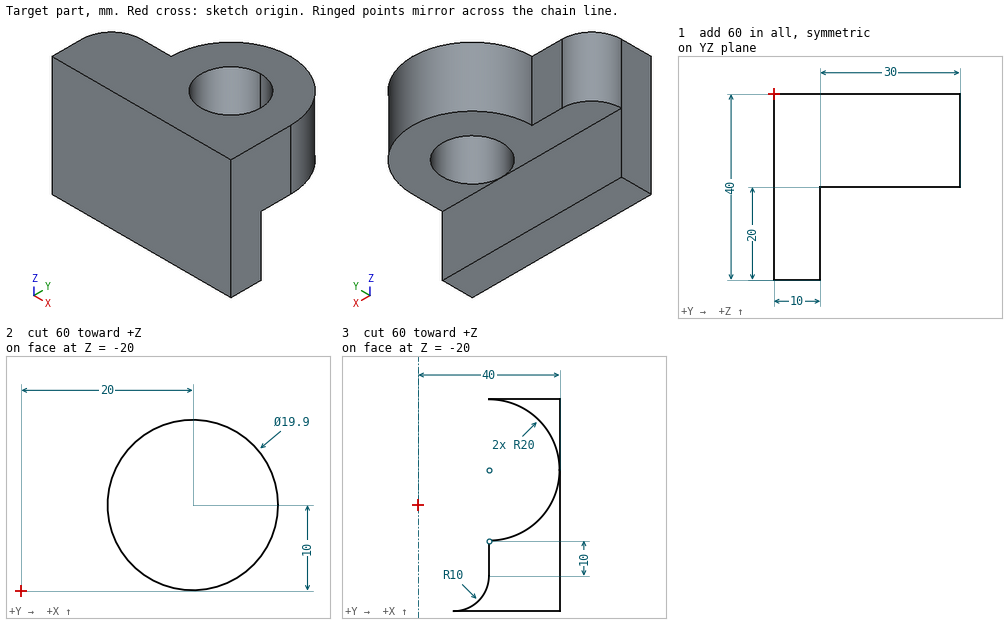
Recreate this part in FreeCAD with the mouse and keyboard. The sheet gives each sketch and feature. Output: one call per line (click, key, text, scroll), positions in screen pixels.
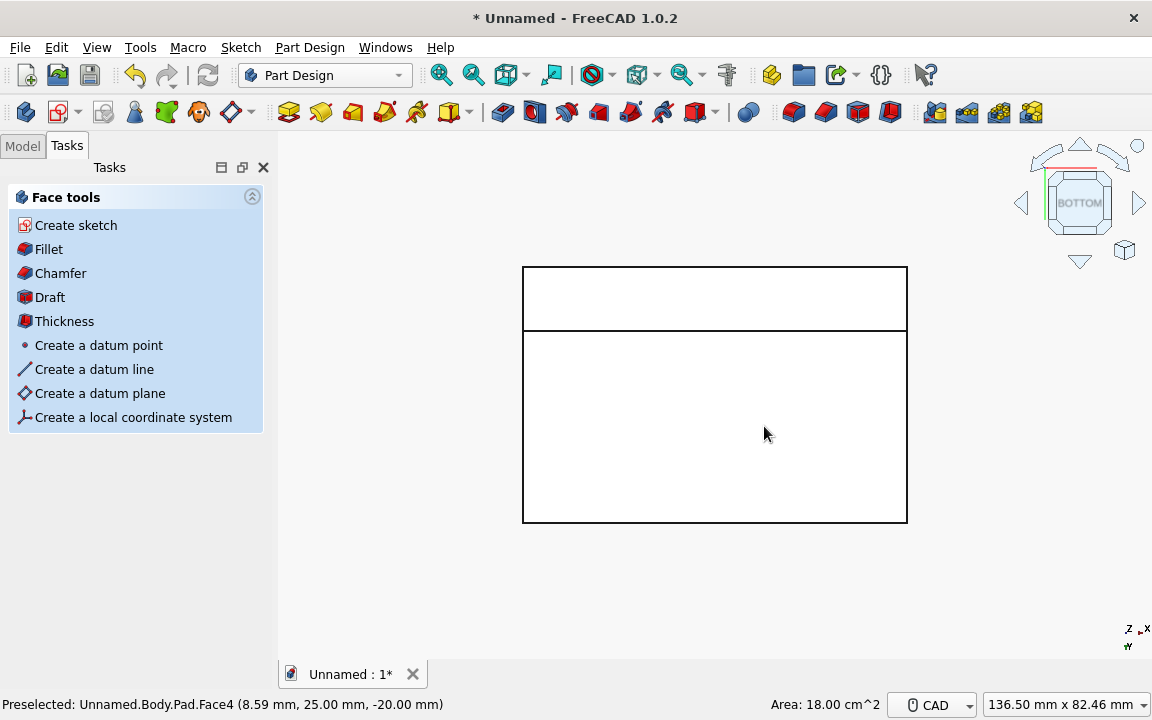
click(58, 112)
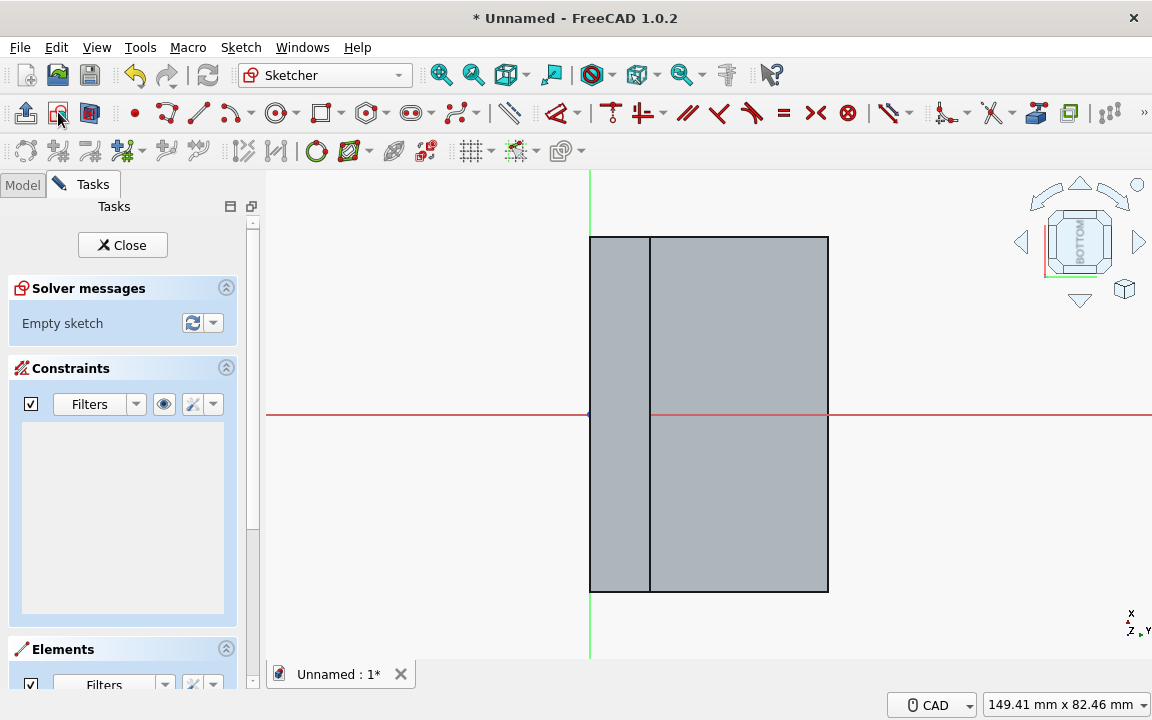
click(90, 114)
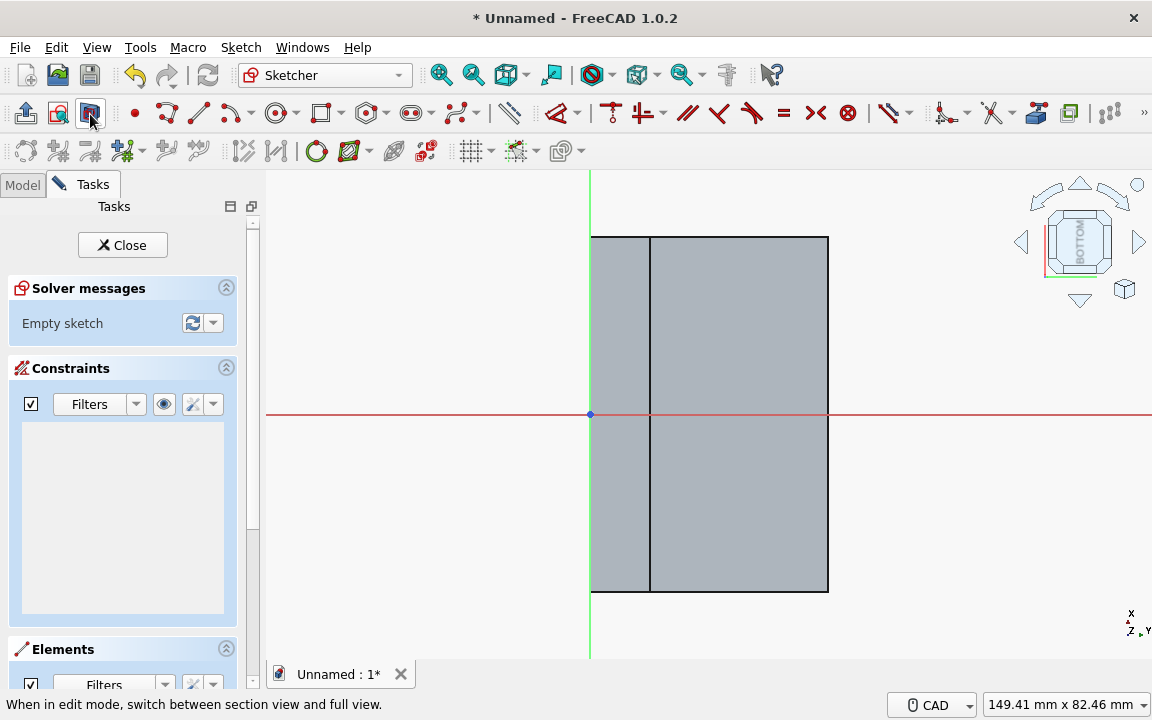
scroll(702, 321, up, 5)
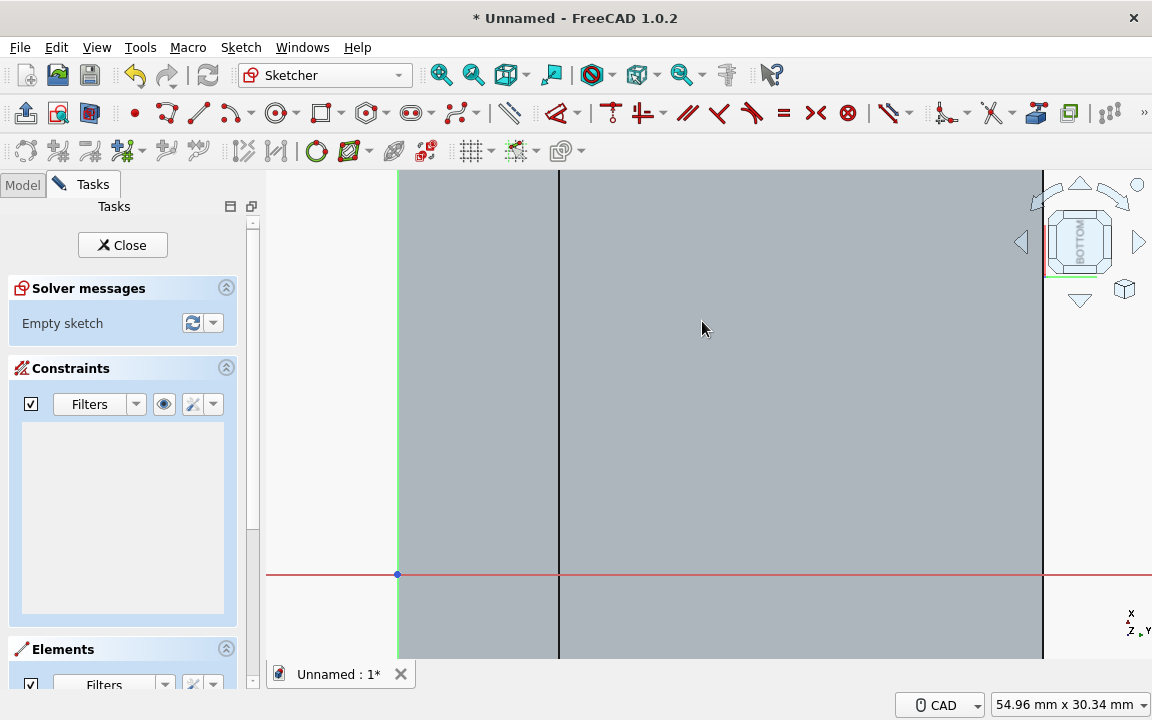
click(276, 114)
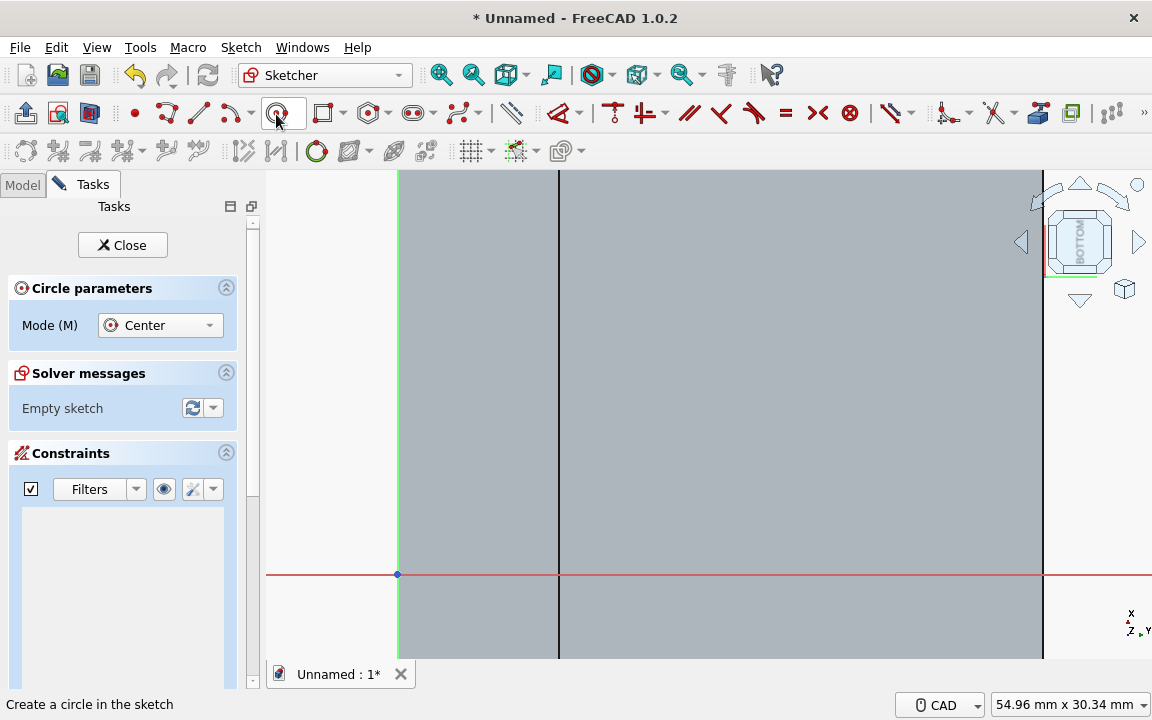
click(720, 413)
move(834, 300)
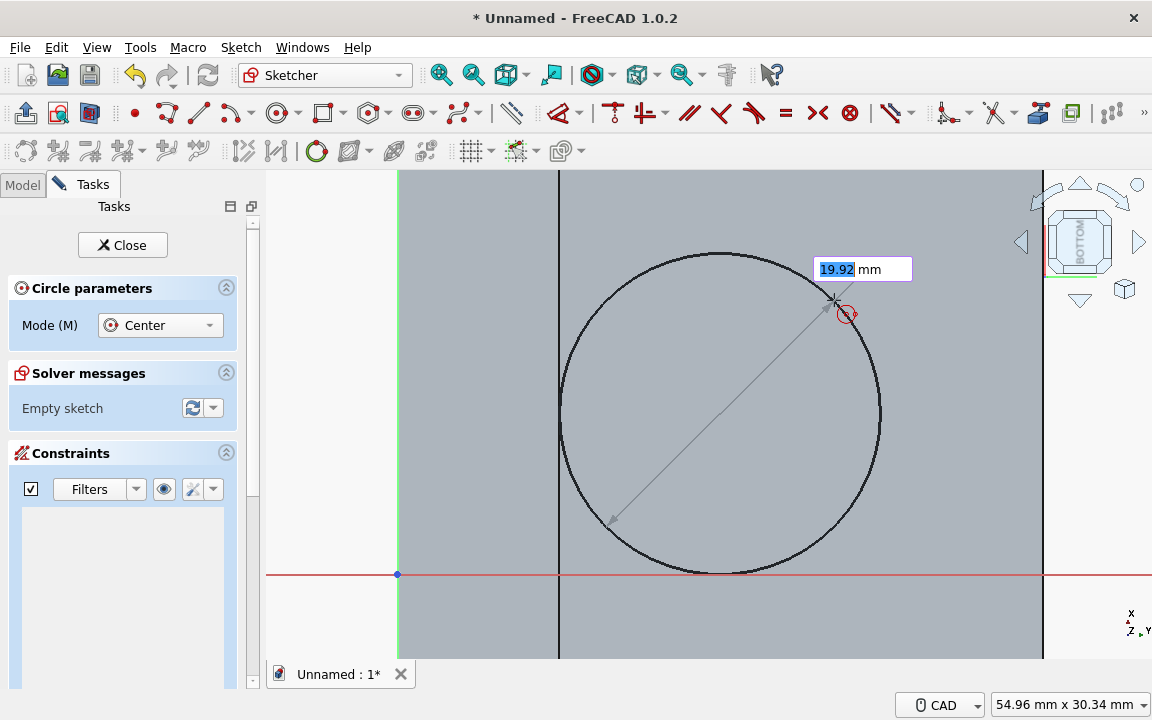
text(19.9)
key(Return)
key(Escape)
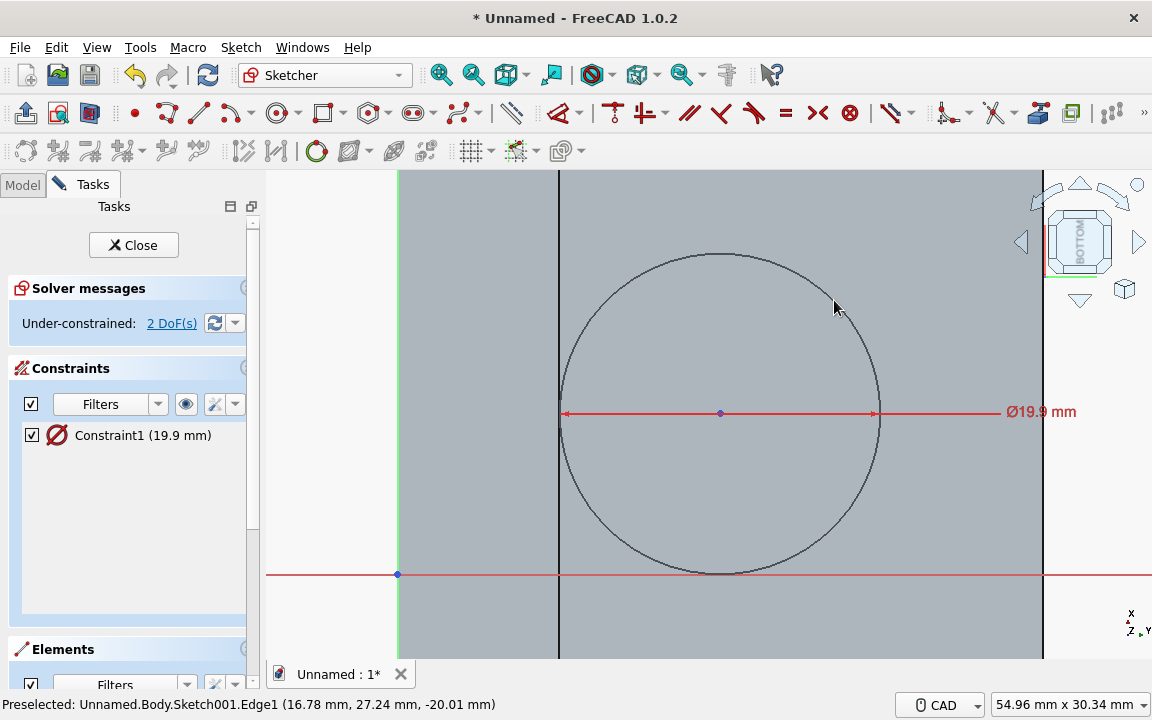
click(558, 114)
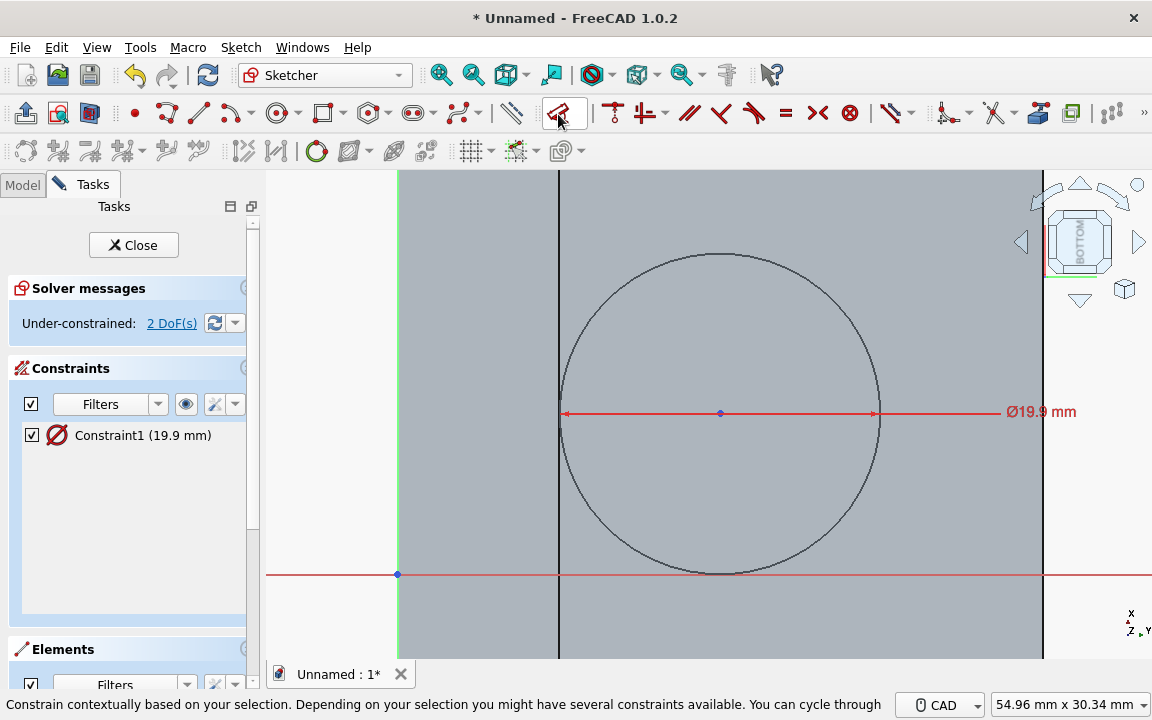
click(720, 414)
click(559, 609)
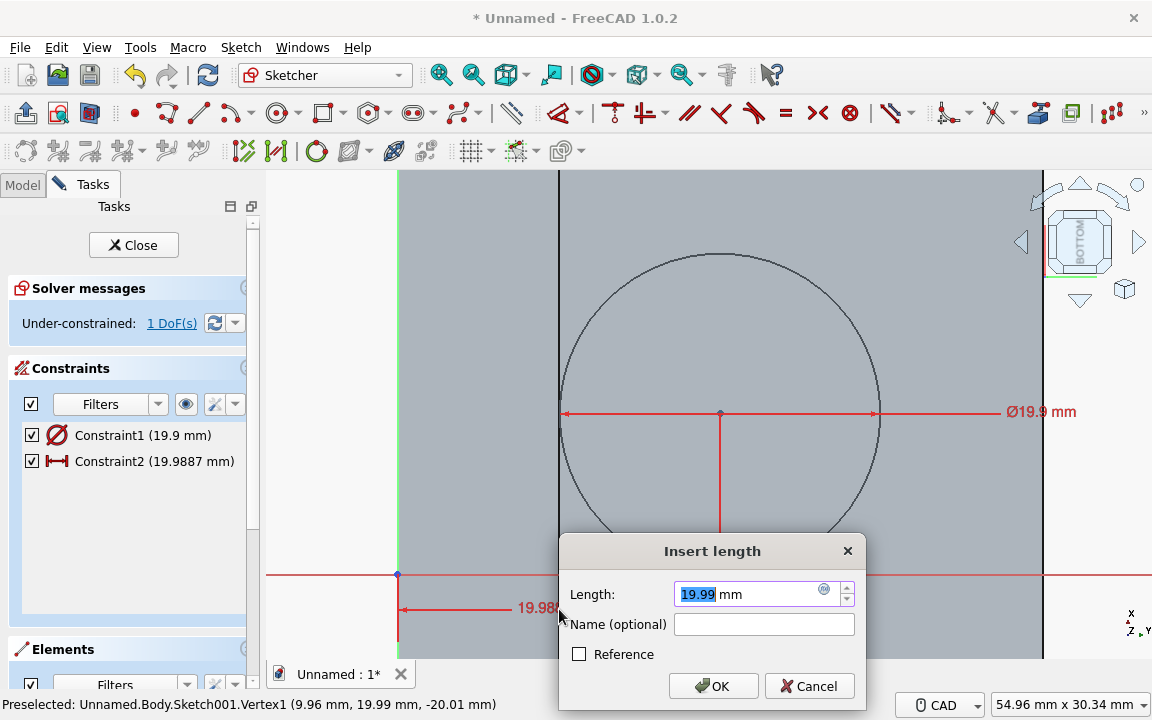
text(20)
key(Return)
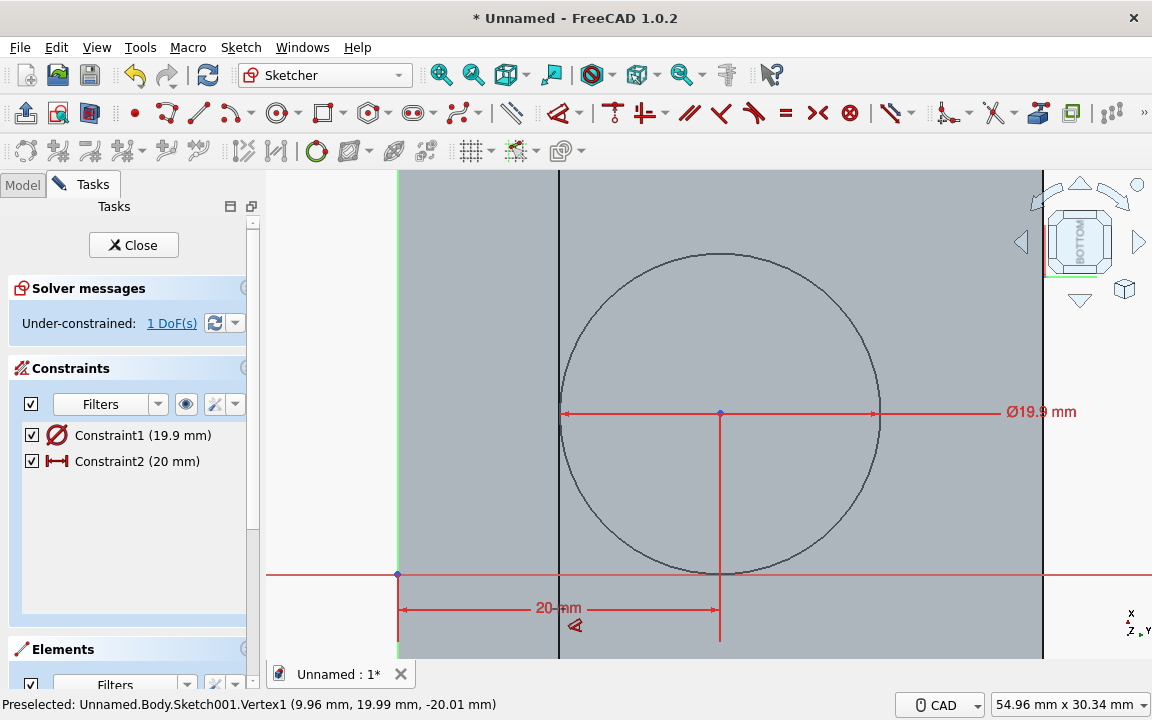
click(720, 414)
click(364, 494)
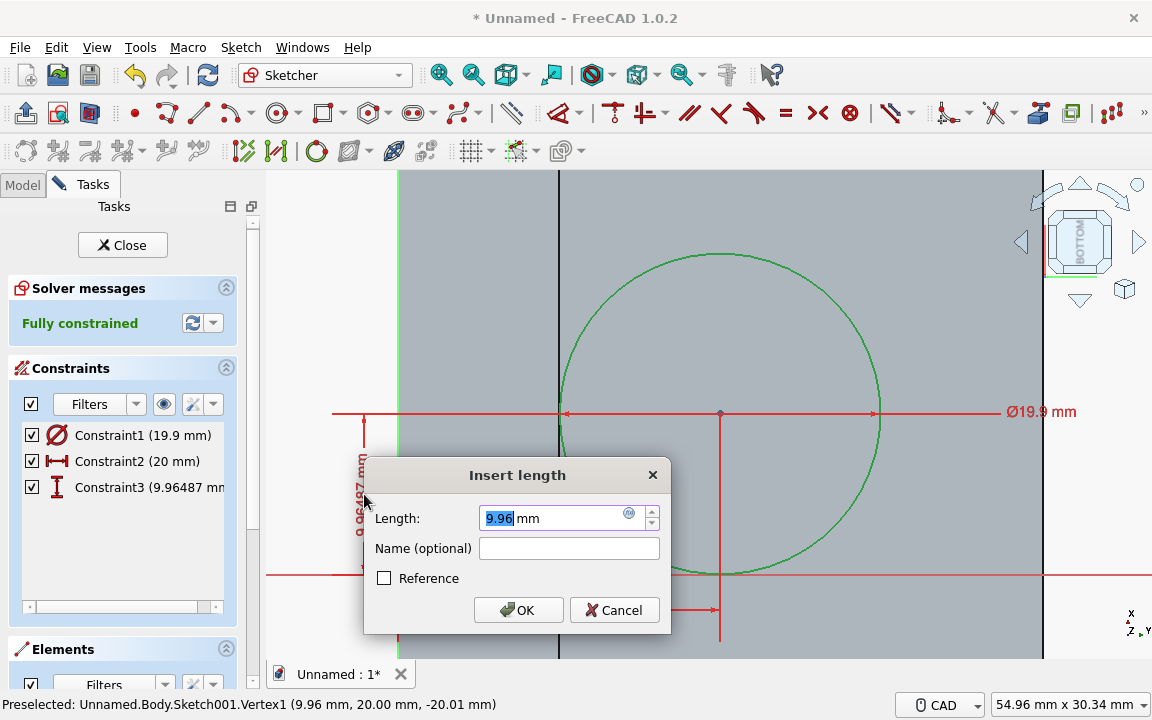
text(10)
key(Return)
key(Escape)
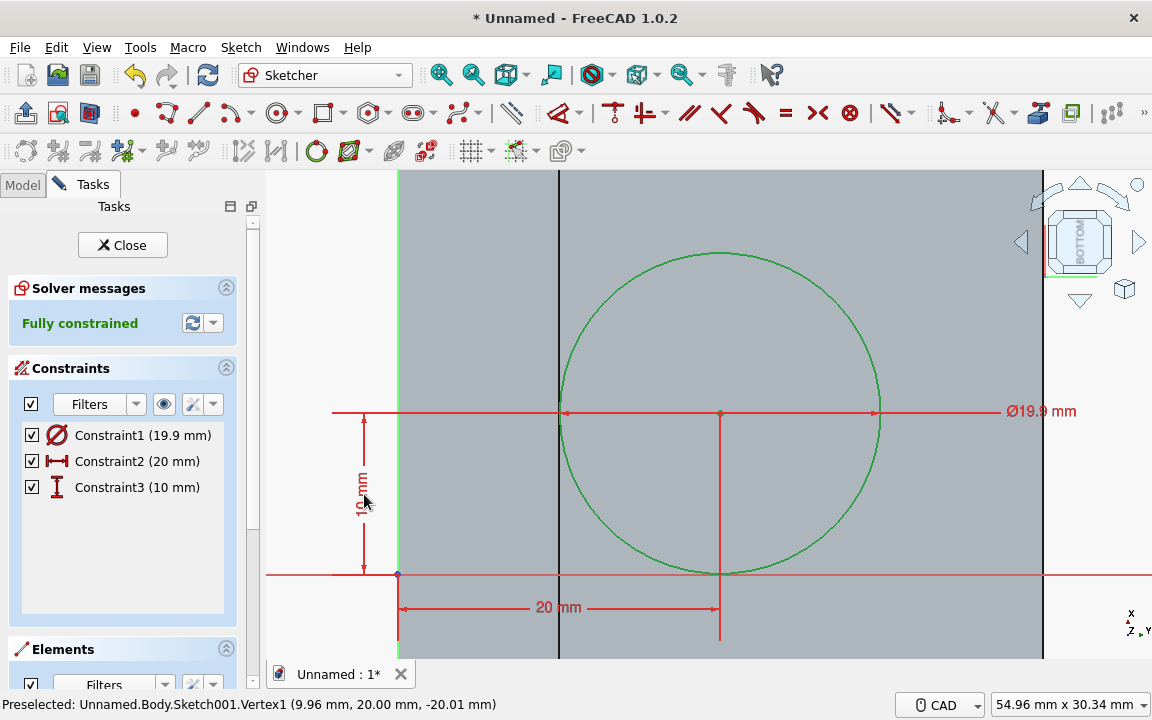
click(123, 245)